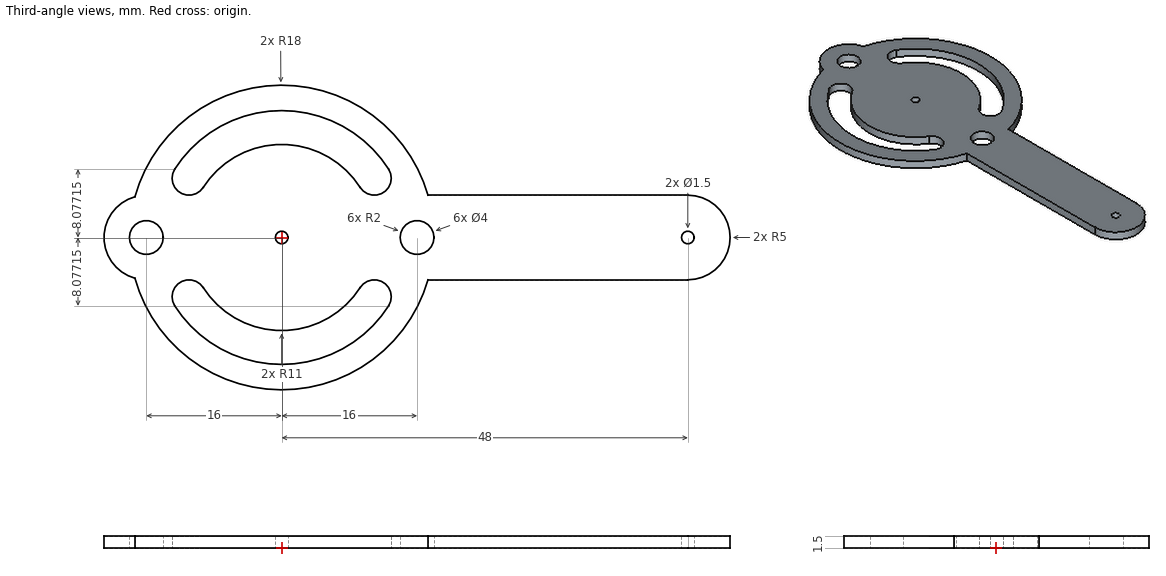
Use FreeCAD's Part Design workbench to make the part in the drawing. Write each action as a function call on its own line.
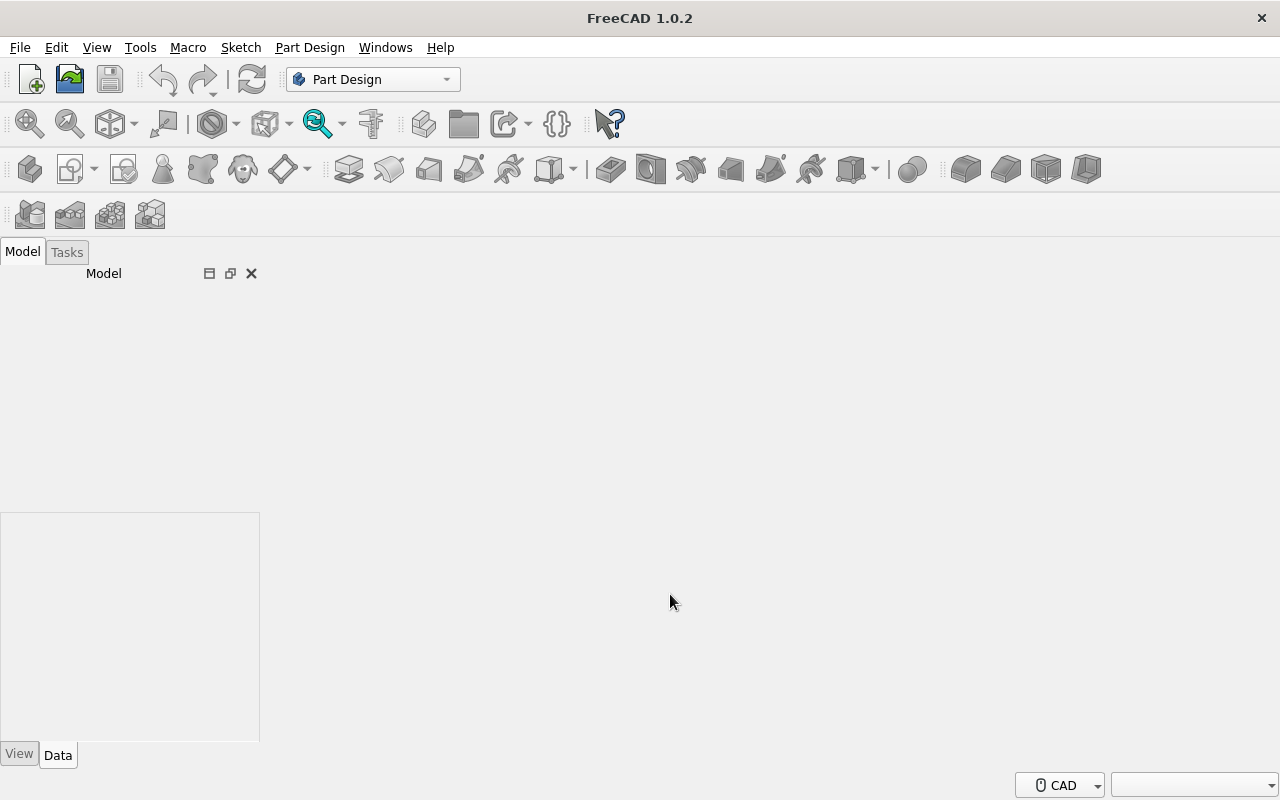
click(30, 80)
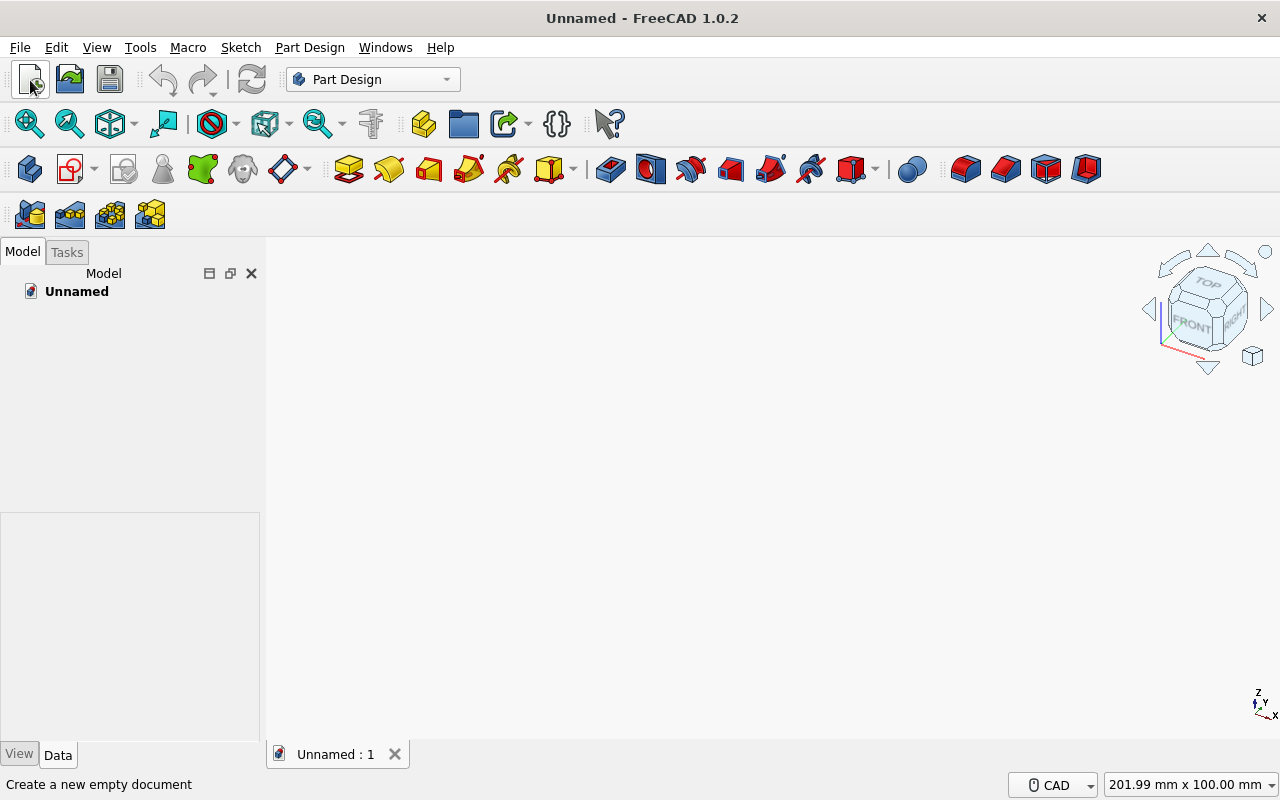
click(70, 170)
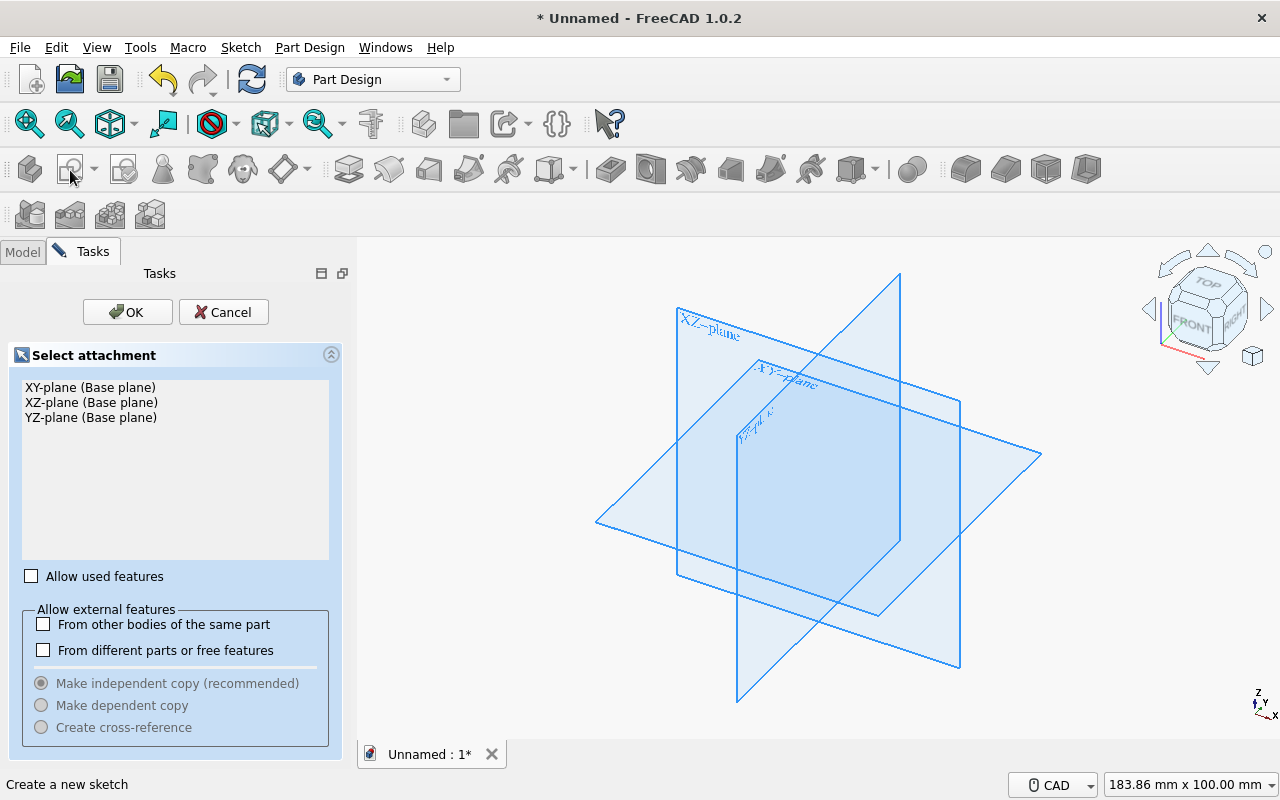
click(82, 388)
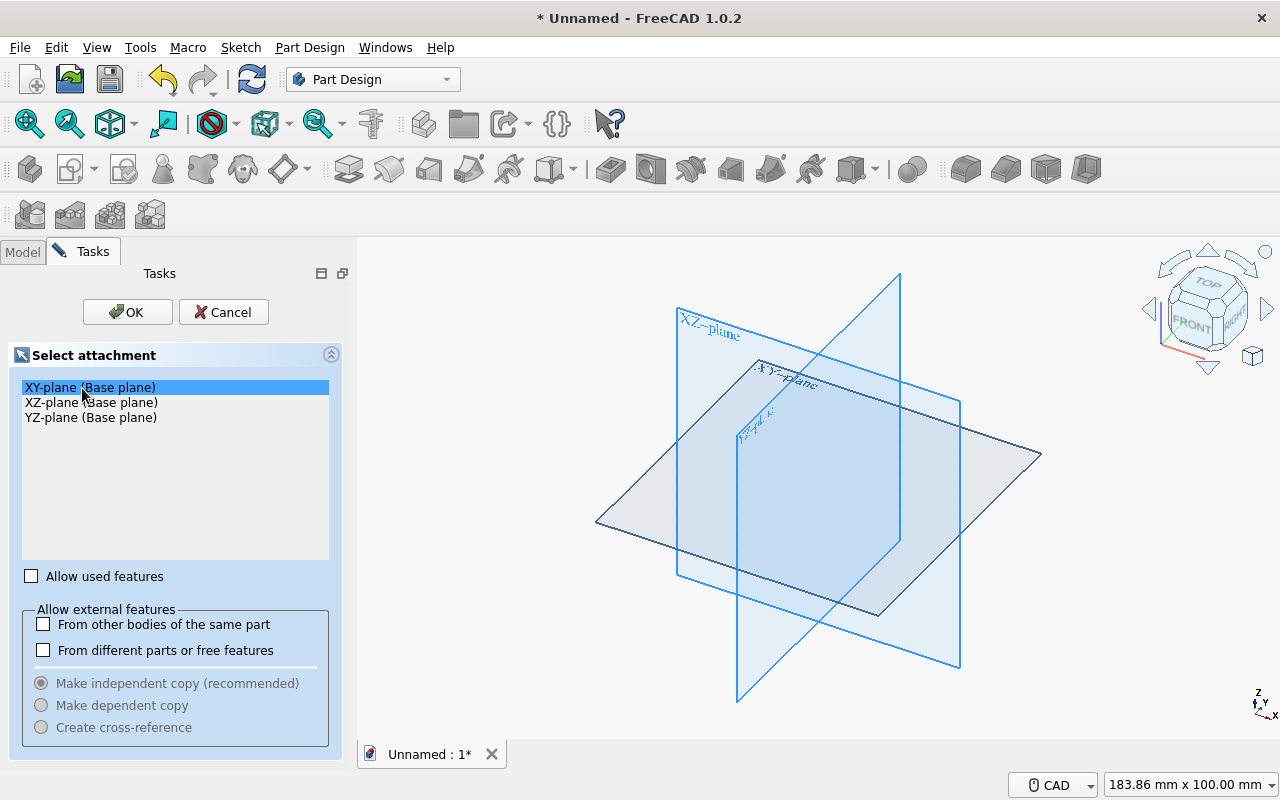
click(128, 312)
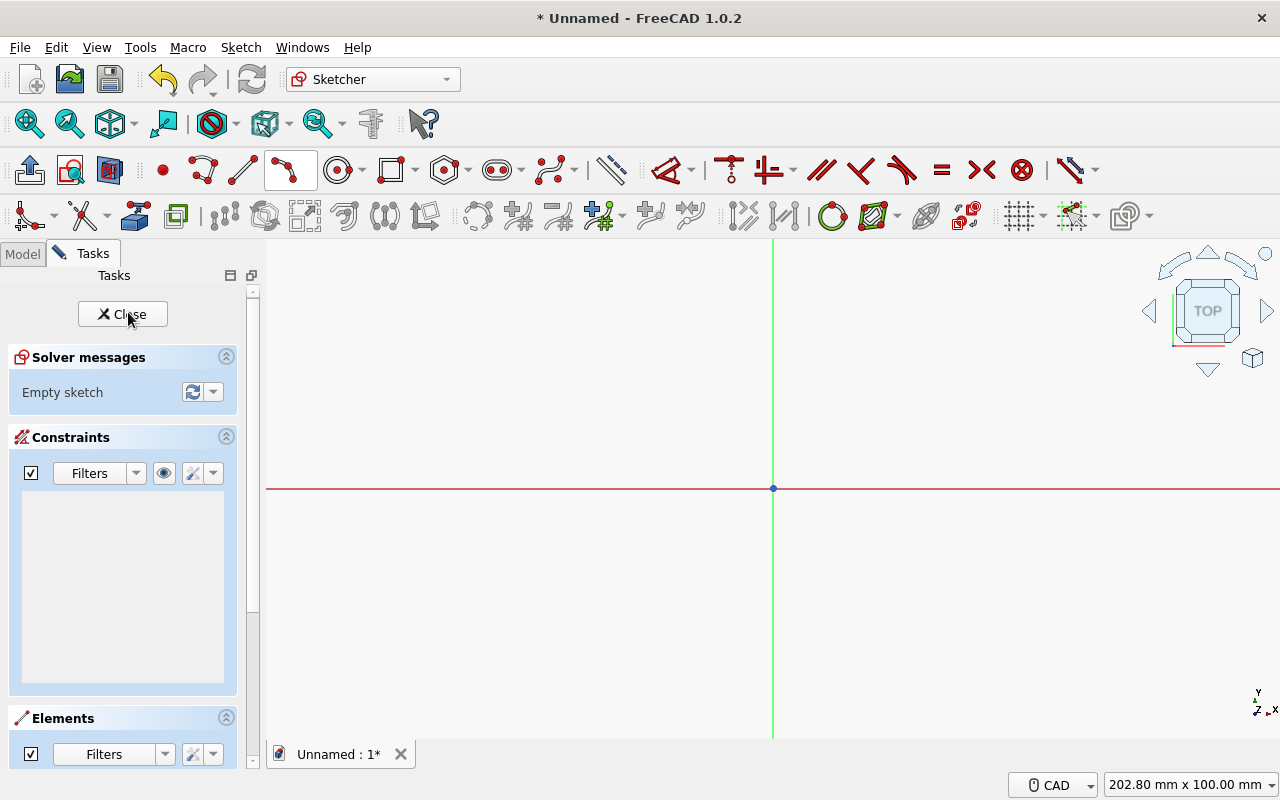
scroll(1115, 489, up, 2)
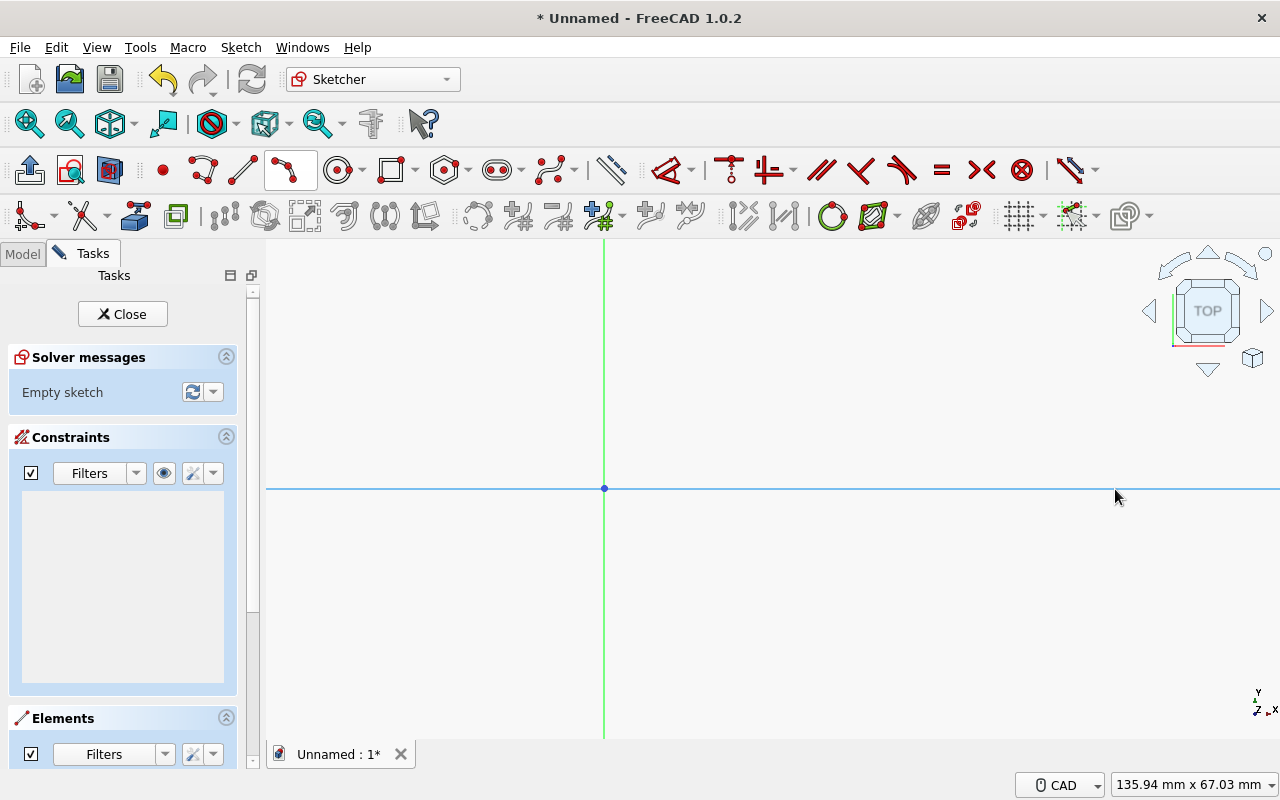
click(244, 170)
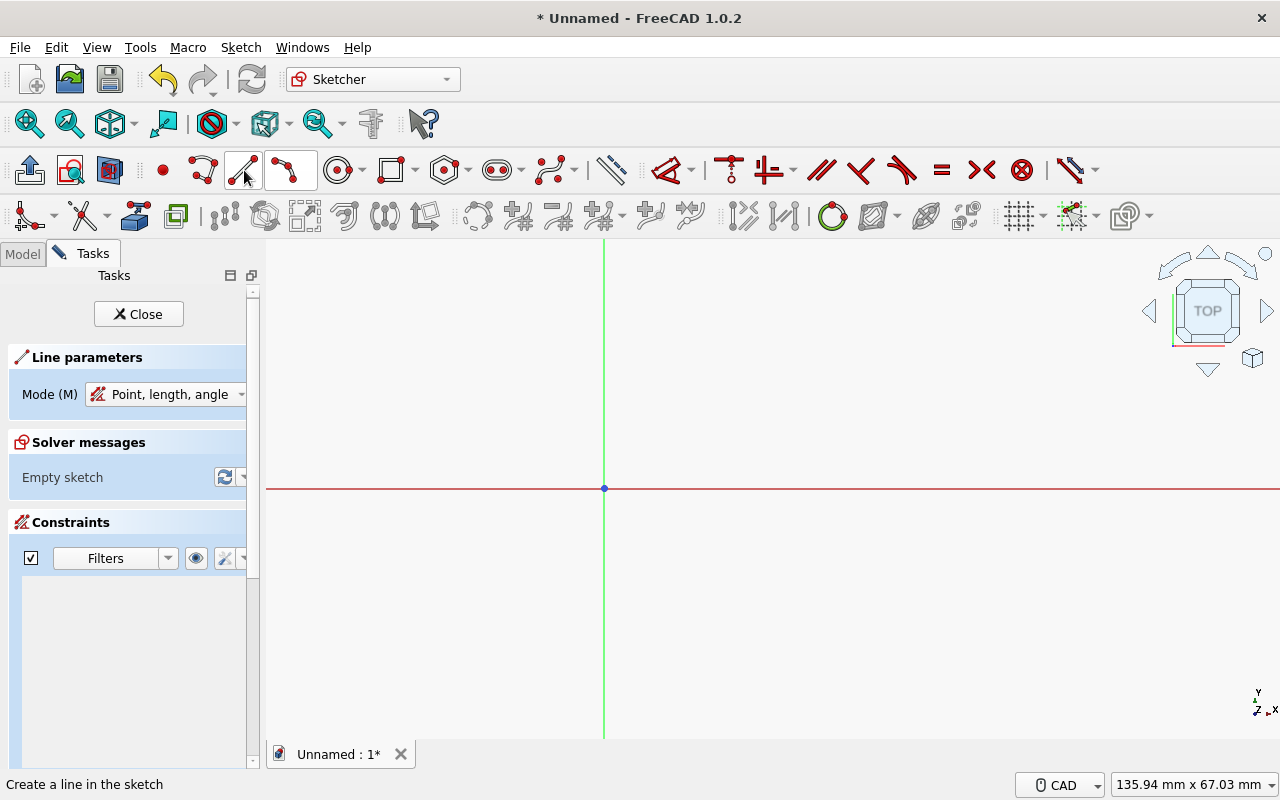
click(733, 526)
click(962, 526)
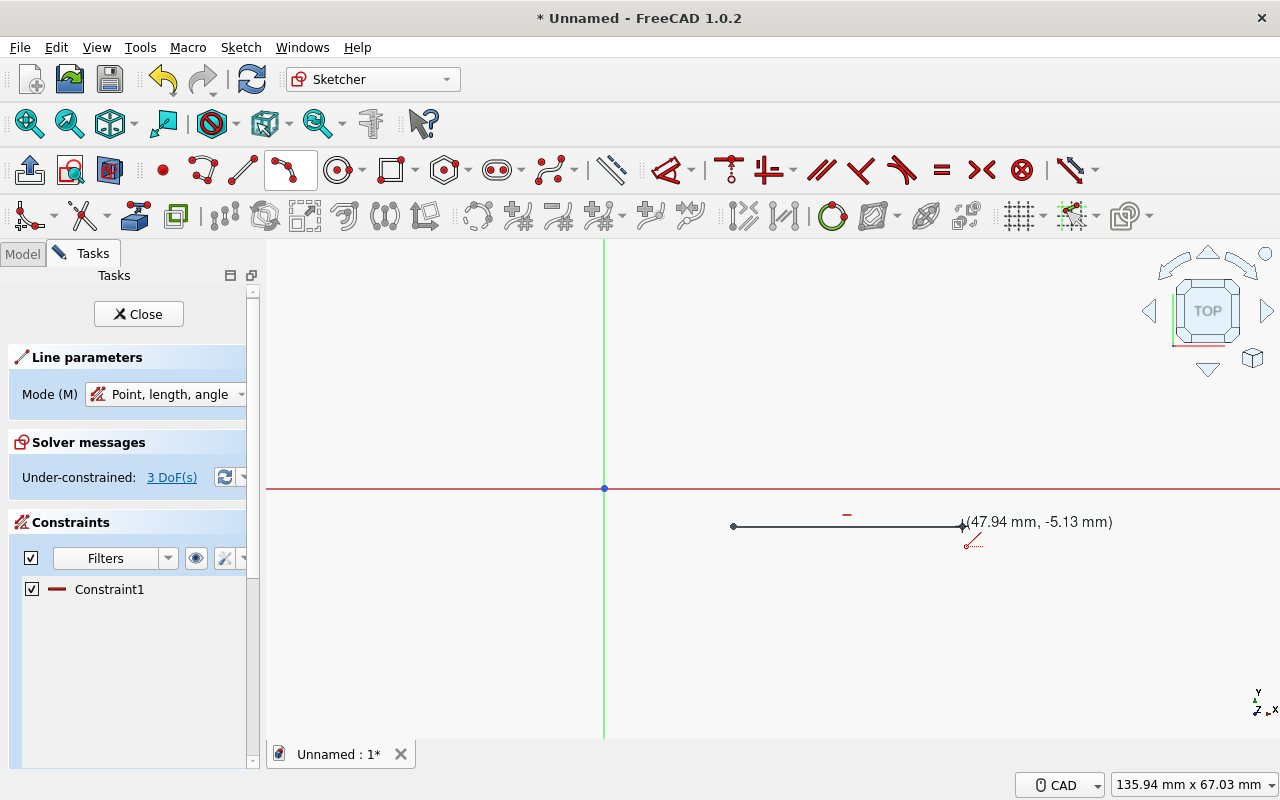
click(962, 451)
click(733, 451)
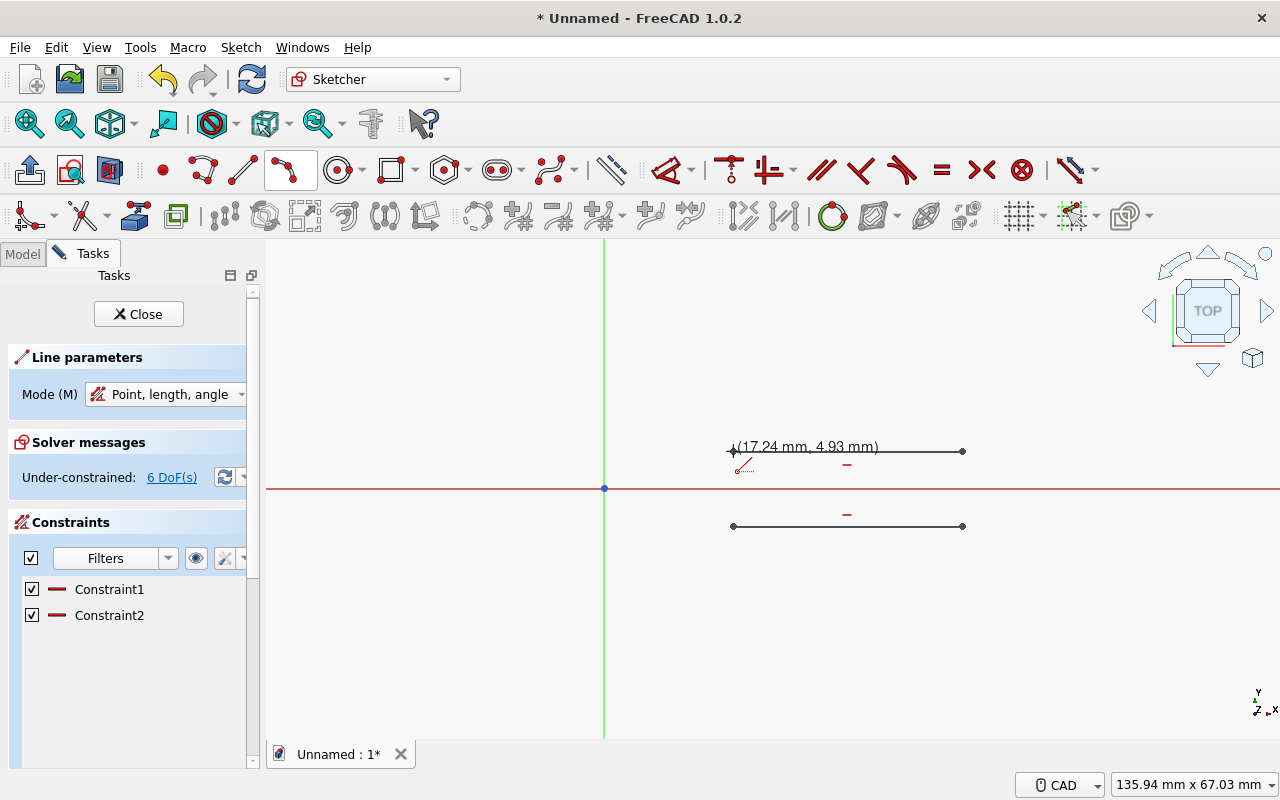
click(284, 170)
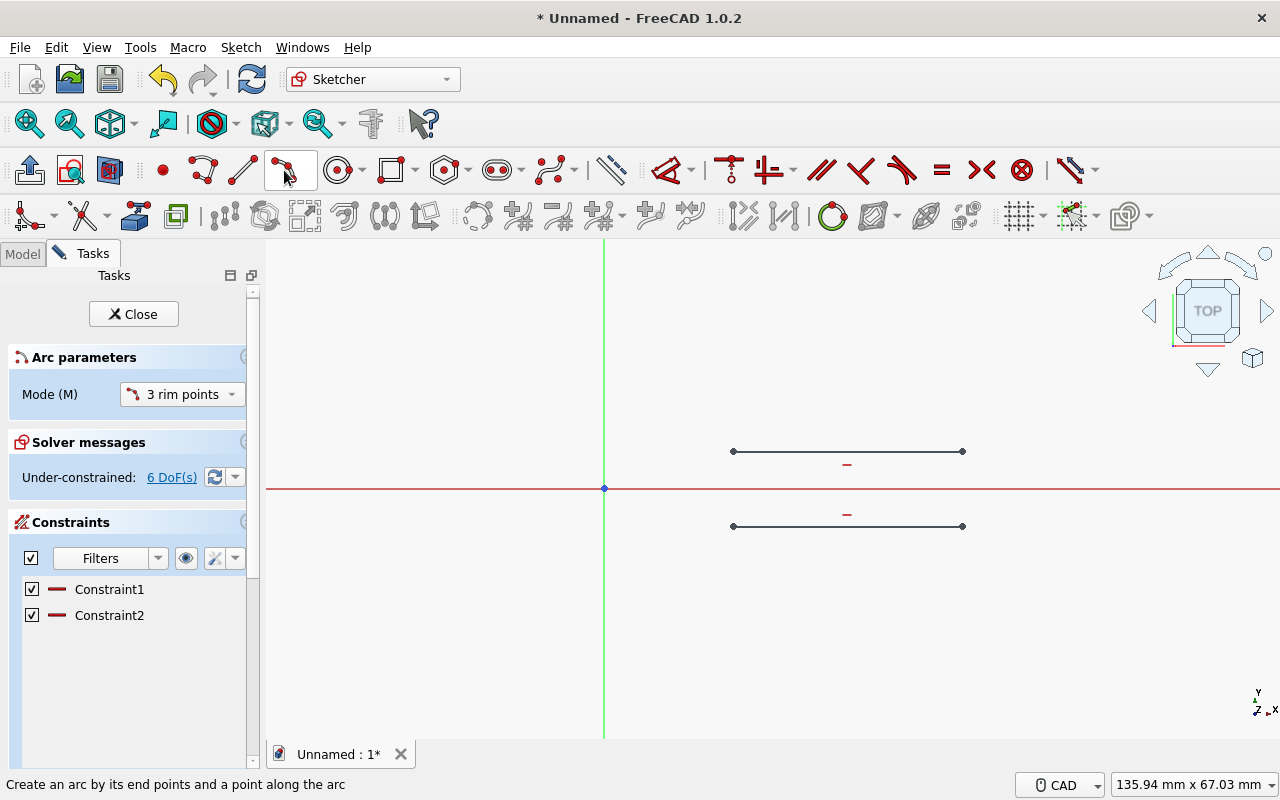
click(962, 527)
click(962, 452)
click(993, 511)